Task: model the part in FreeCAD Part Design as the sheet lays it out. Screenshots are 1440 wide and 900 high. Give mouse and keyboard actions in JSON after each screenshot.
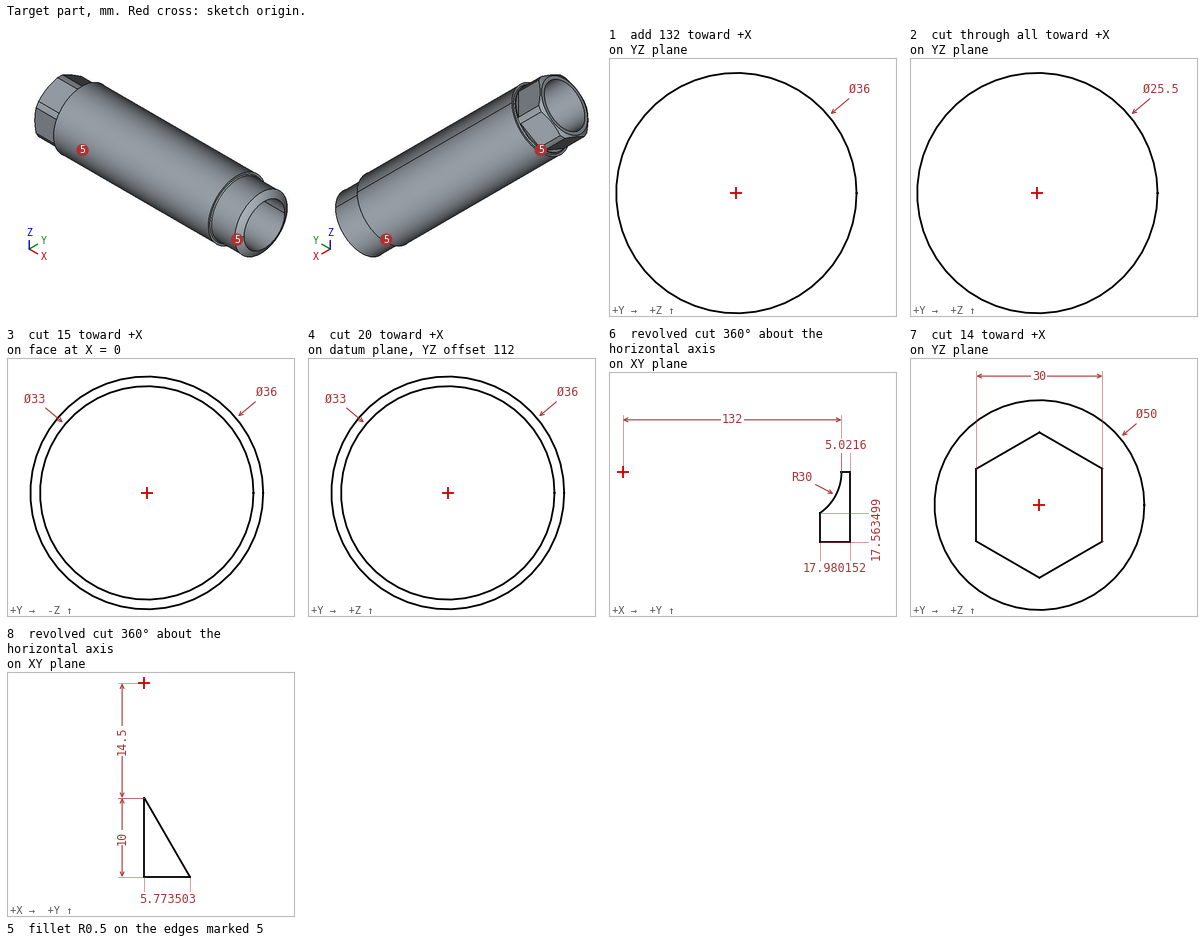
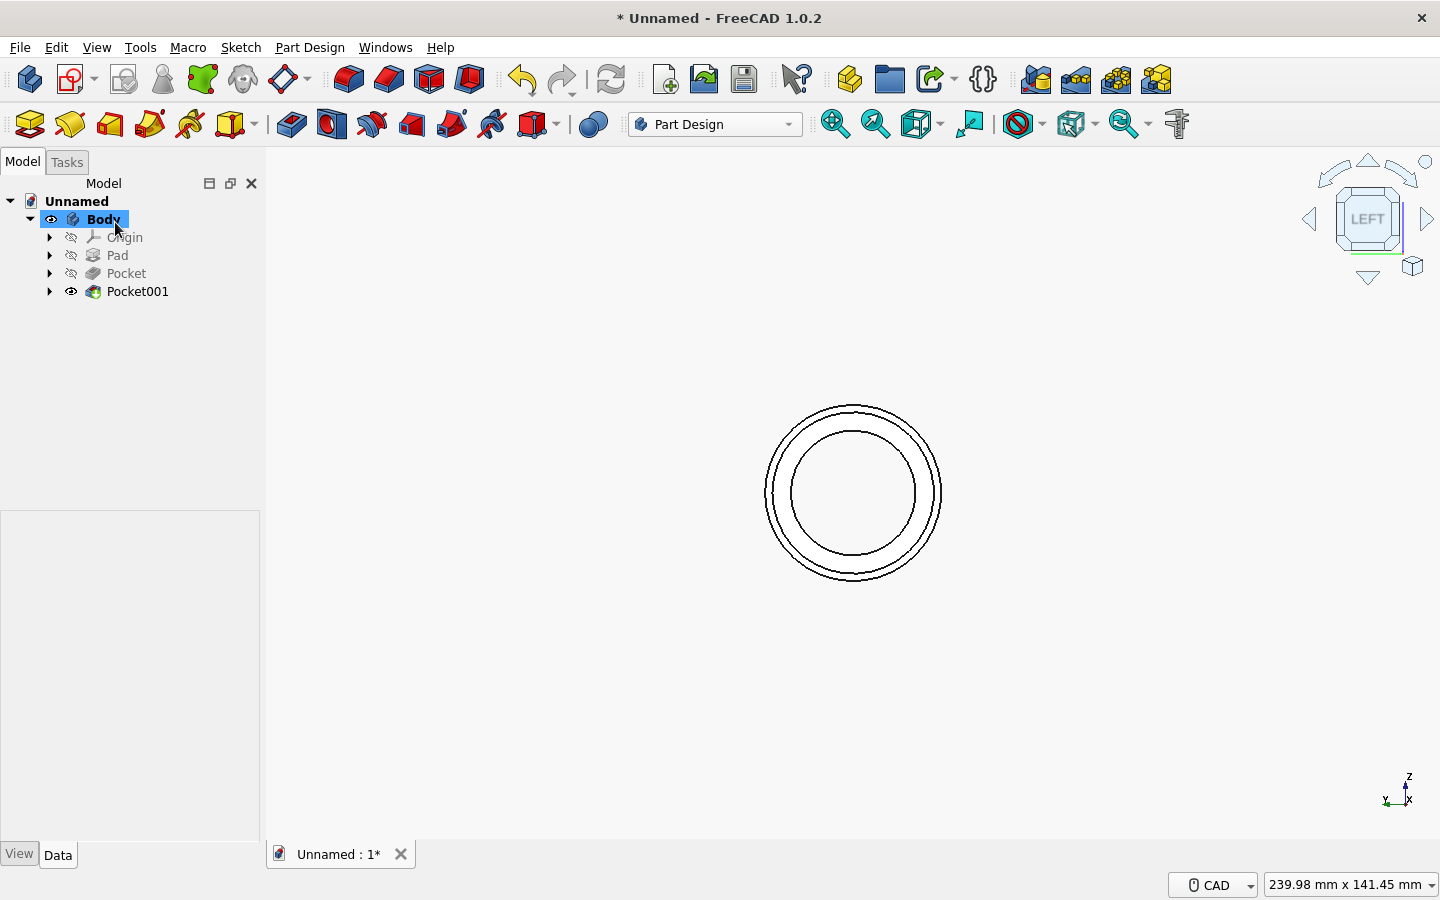
{"action": "left_click", "coordinate": [50, 237]}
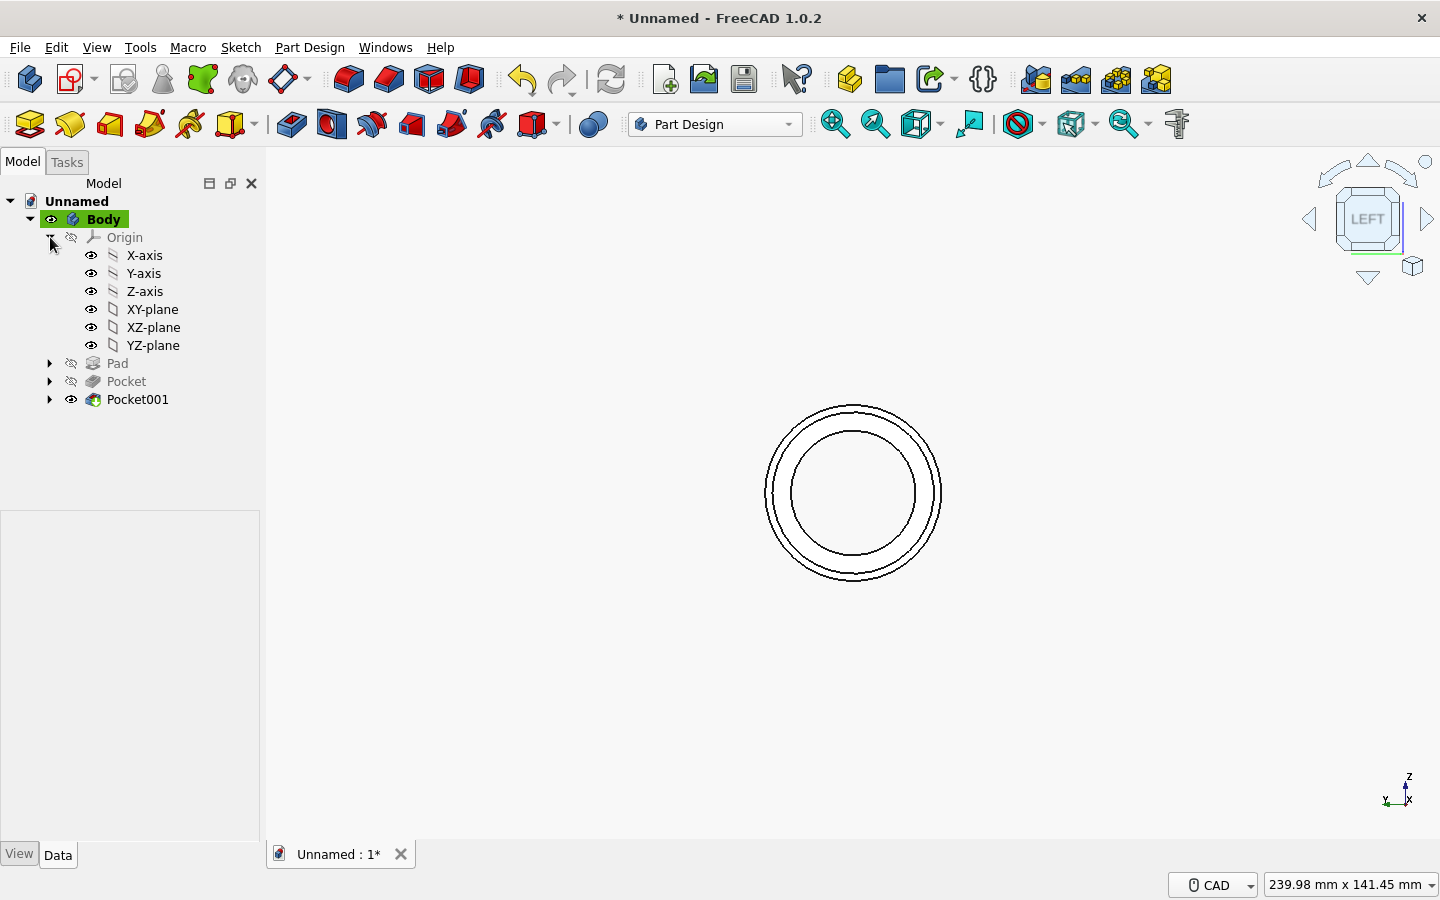
{"action": "left_click", "coordinate": [136, 345]}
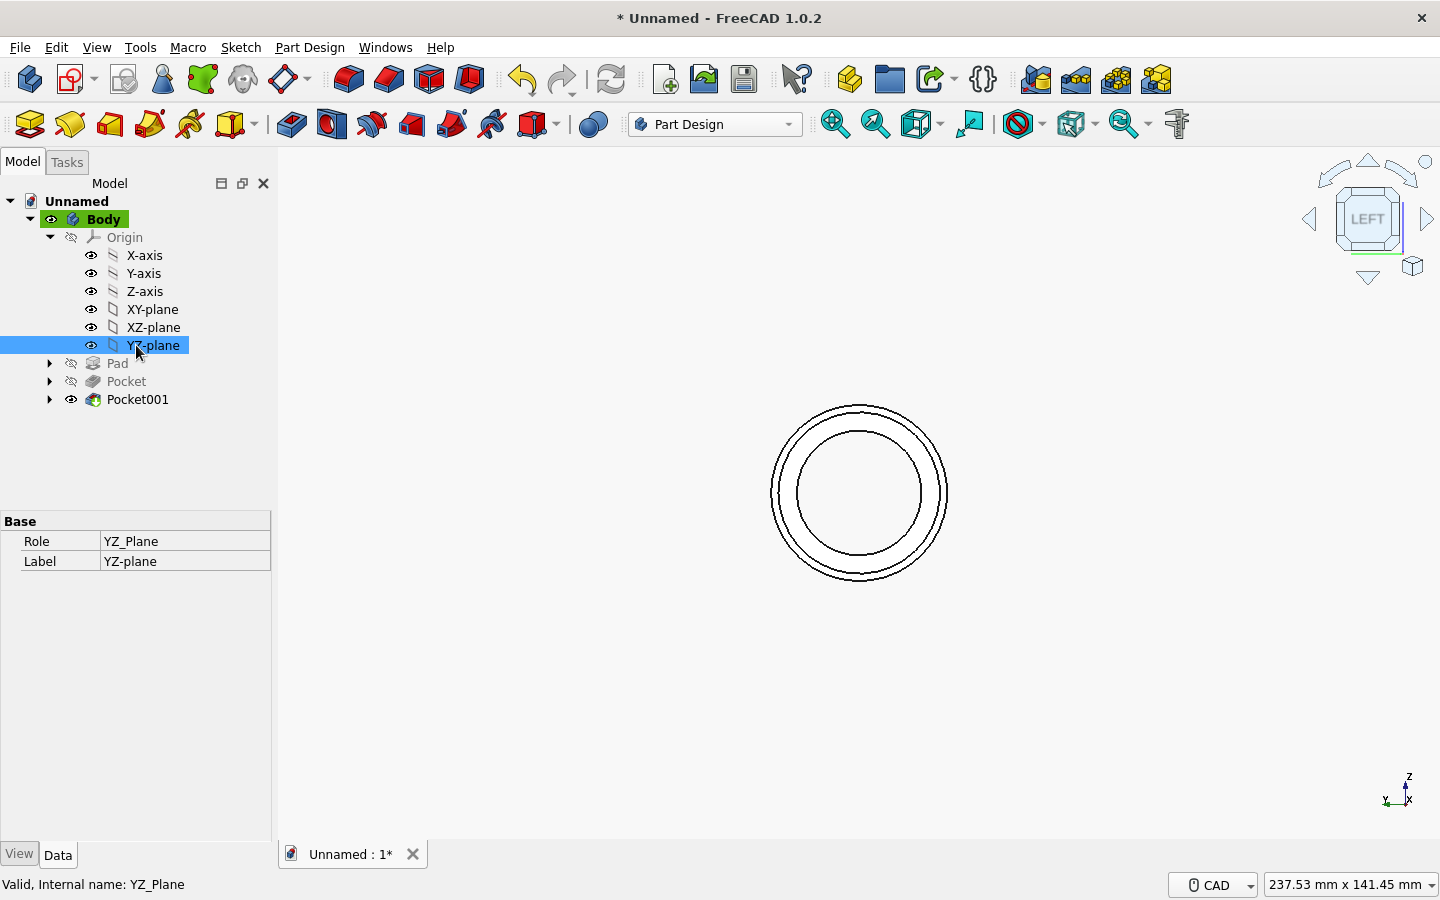
{"action": "left_click", "coordinate": [284, 80]}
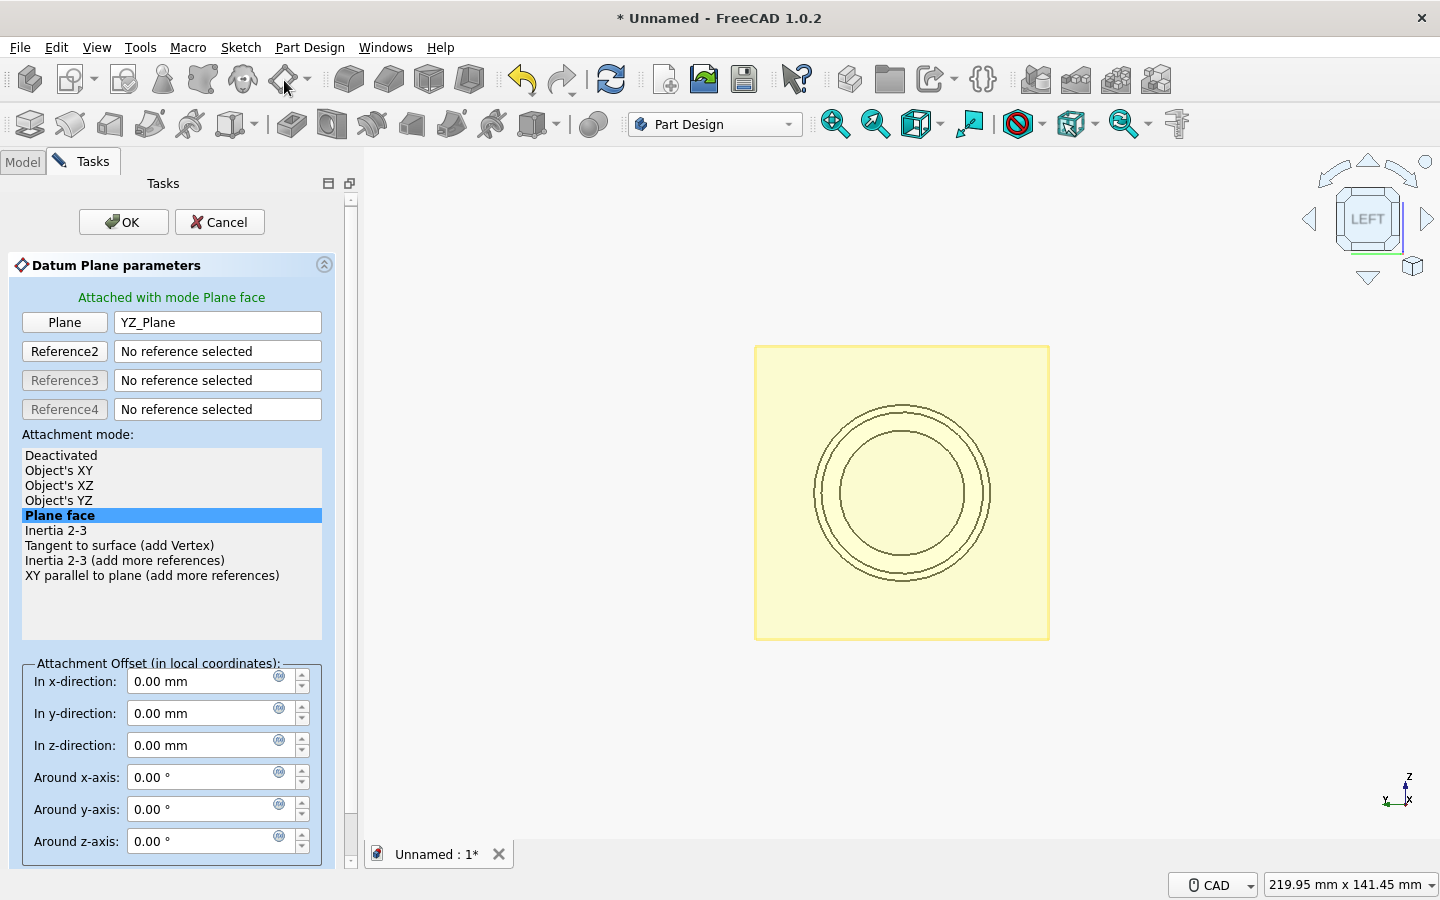
{"action": "triple_click", "coordinate": [210, 745]}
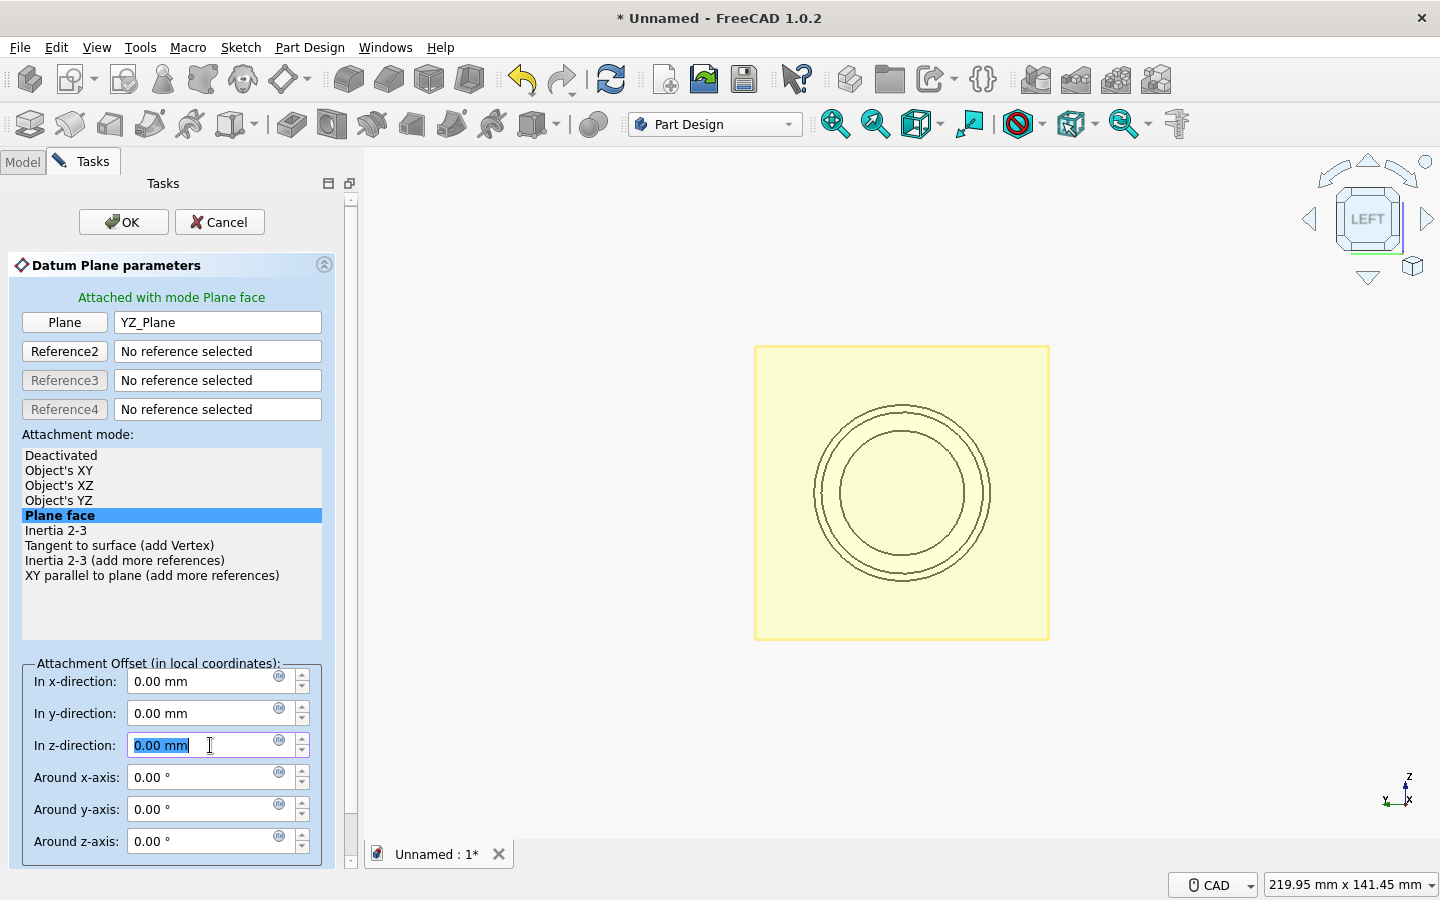
{"action": "type", "text": "112"}
{"action": "key", "text": "Tab"}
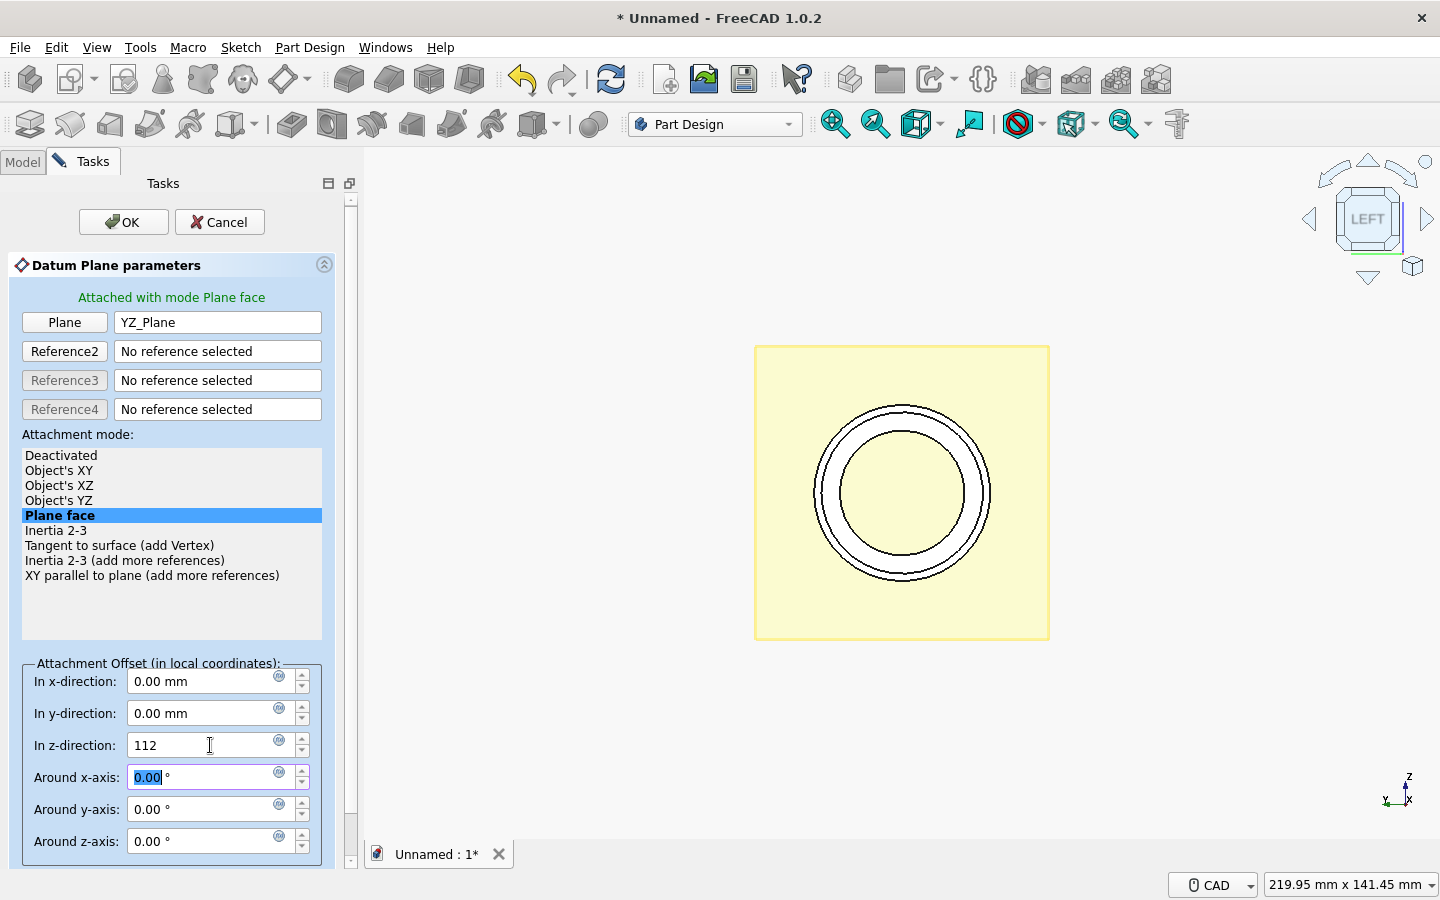
{"action": "left_click", "coordinate": [124, 222]}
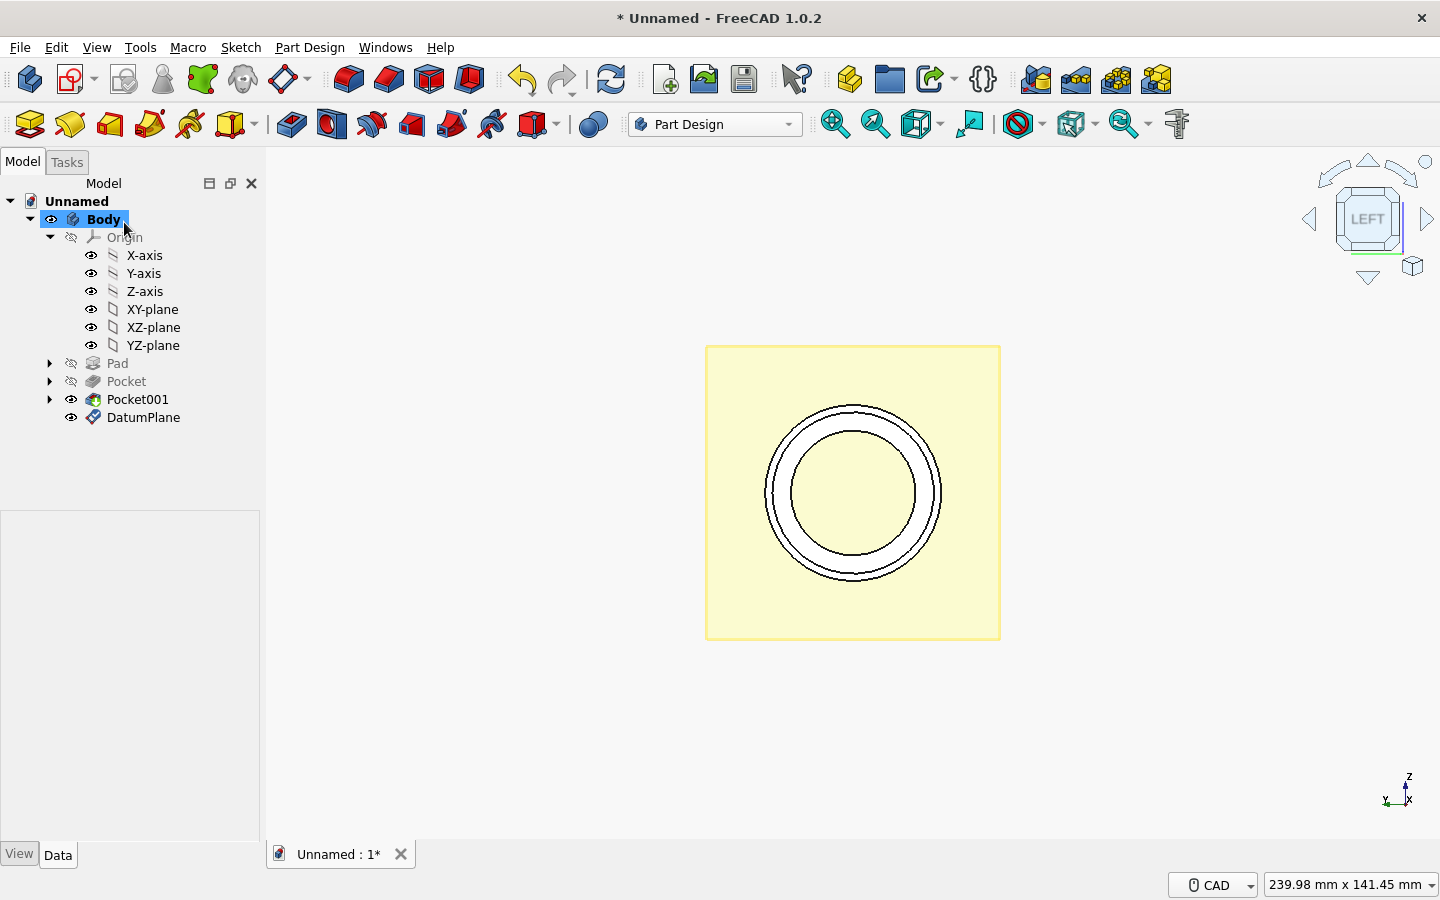
{"action": "left_click", "coordinate": [116, 417]}